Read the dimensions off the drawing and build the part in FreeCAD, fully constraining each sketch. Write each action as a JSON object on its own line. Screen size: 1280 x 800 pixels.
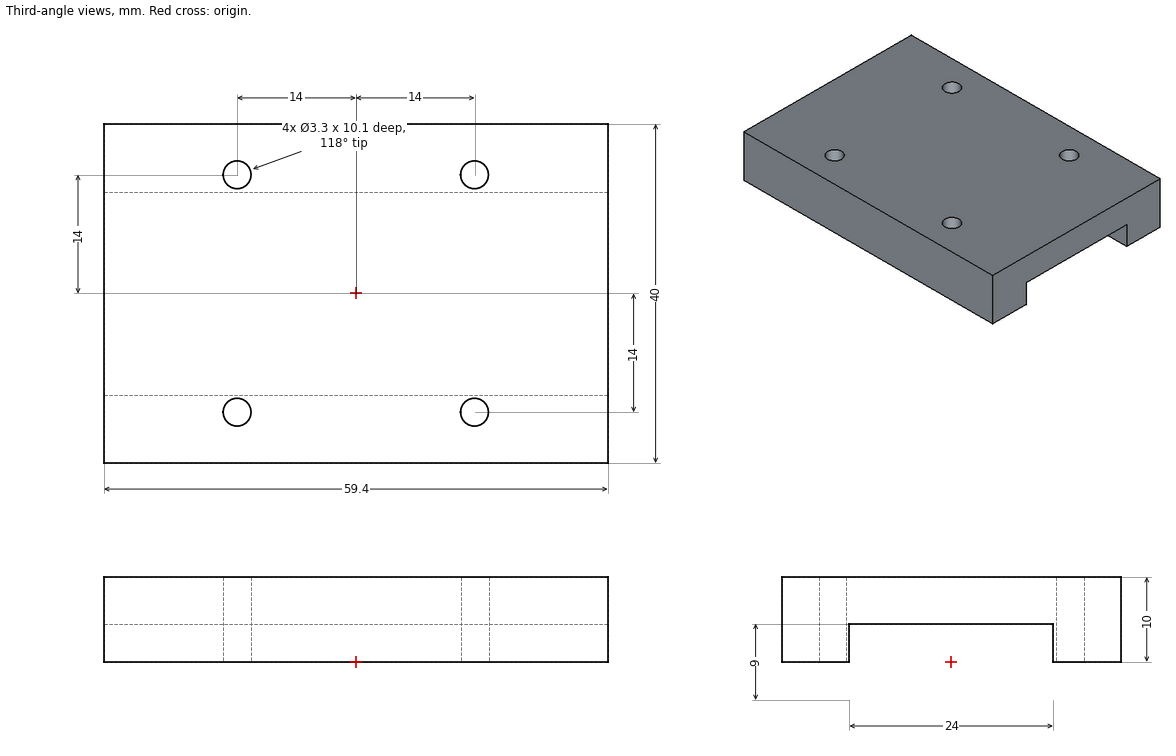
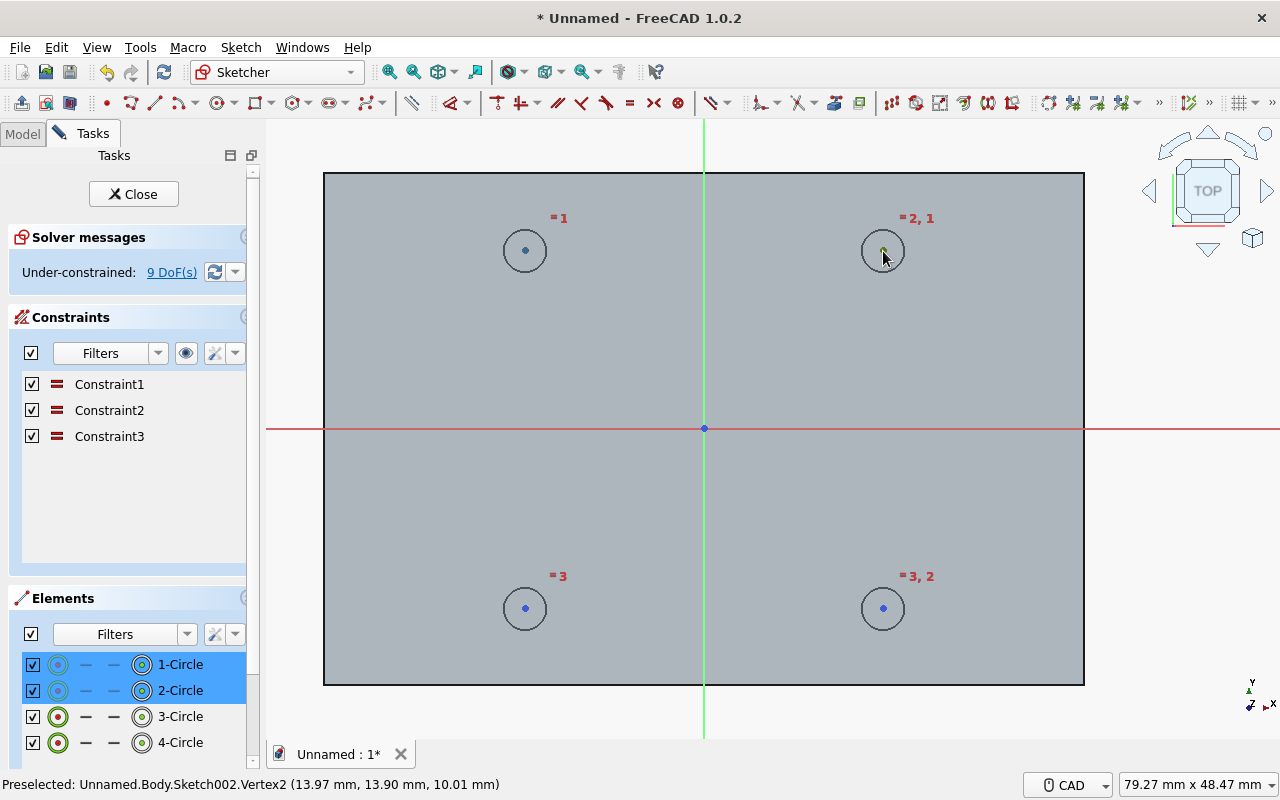
{"action": "key", "text": "h"}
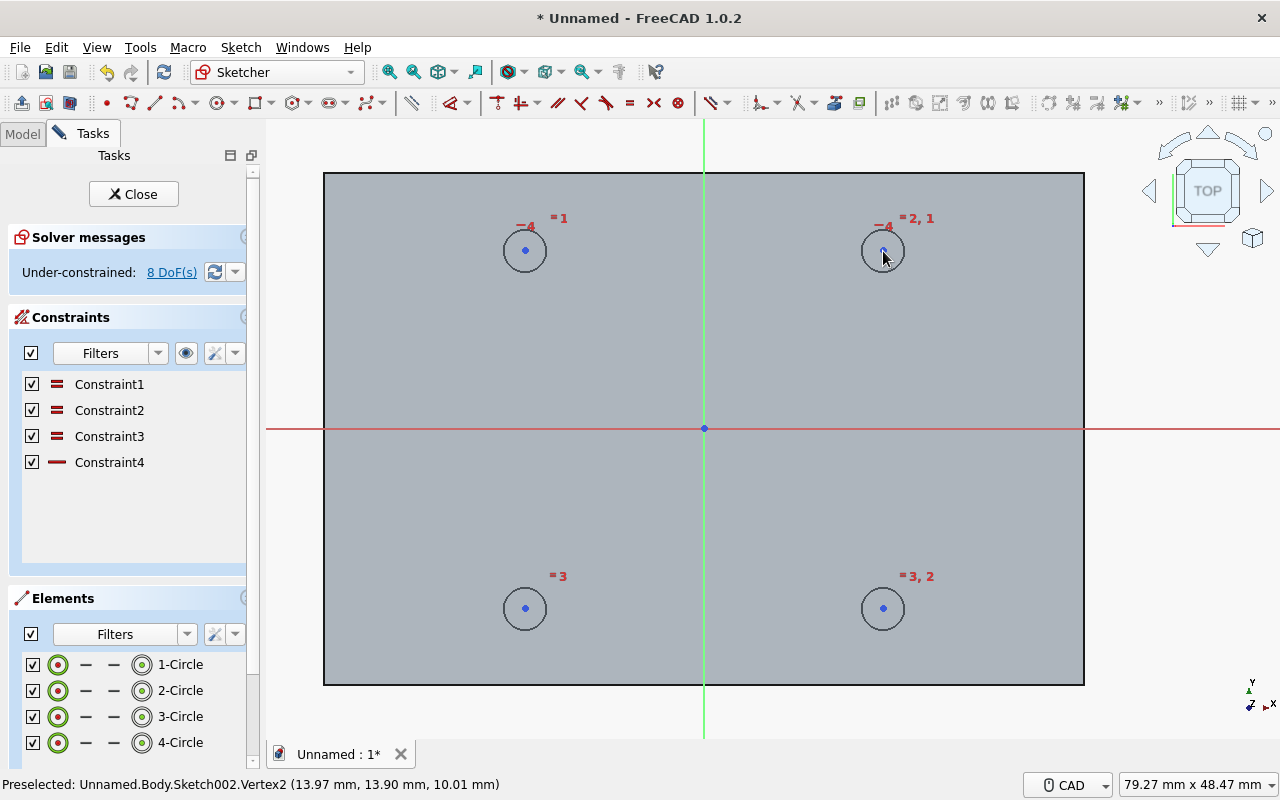
{"action": "left_click", "coordinate": [883, 251]}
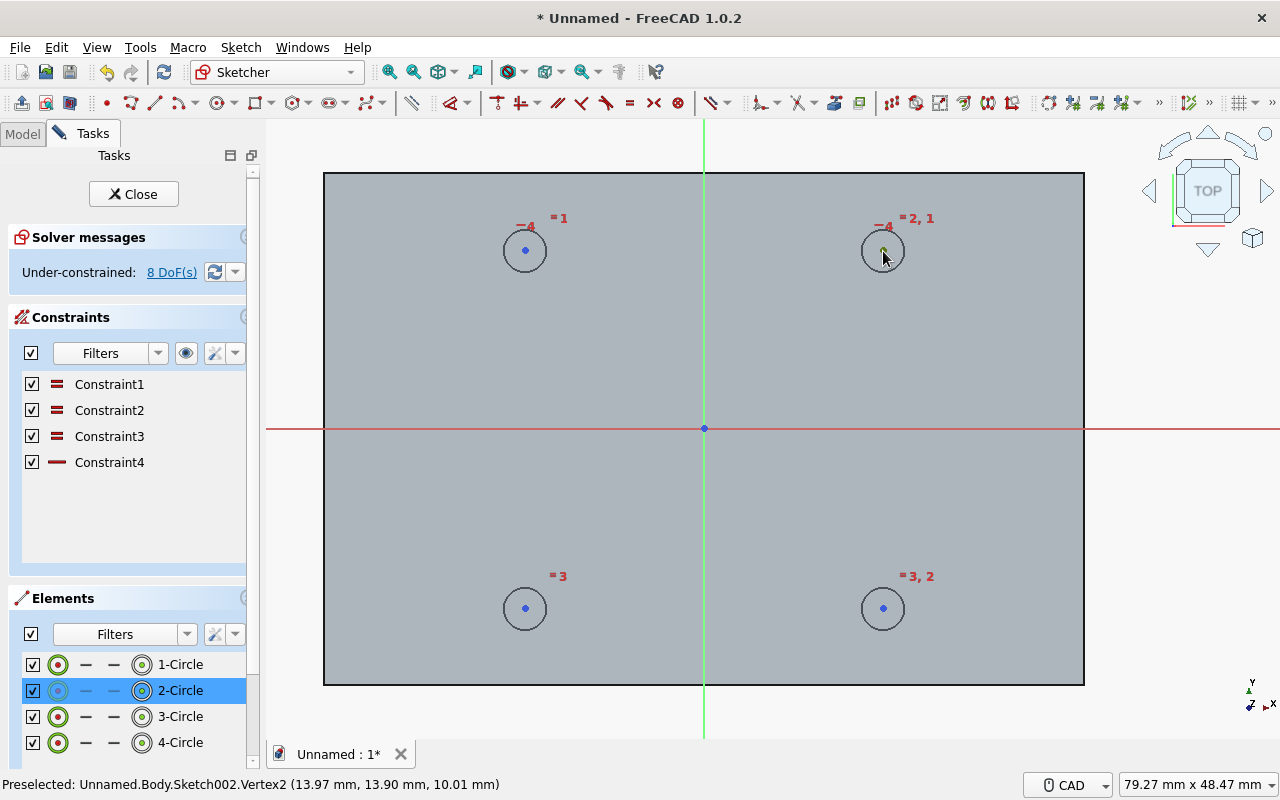
{"action": "left_click", "coordinate": [883, 609]}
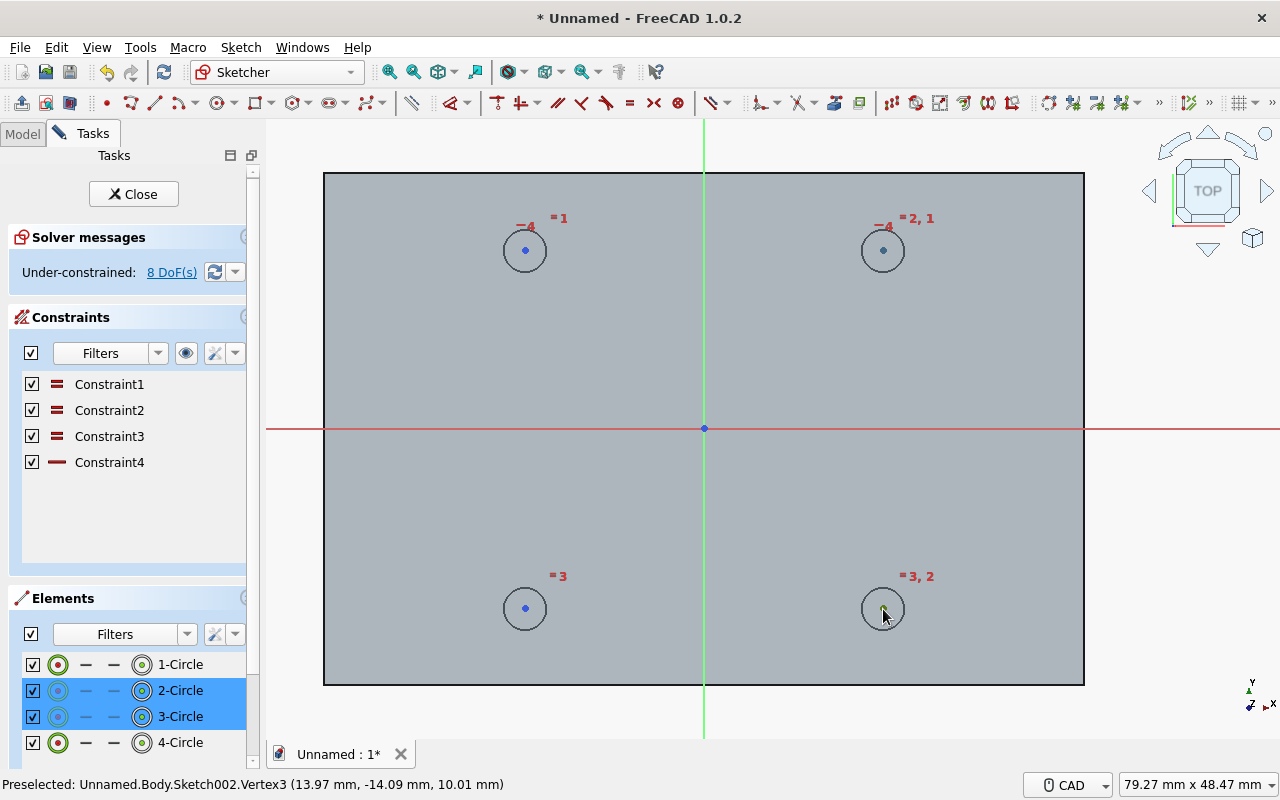
{"action": "key", "text": "v"}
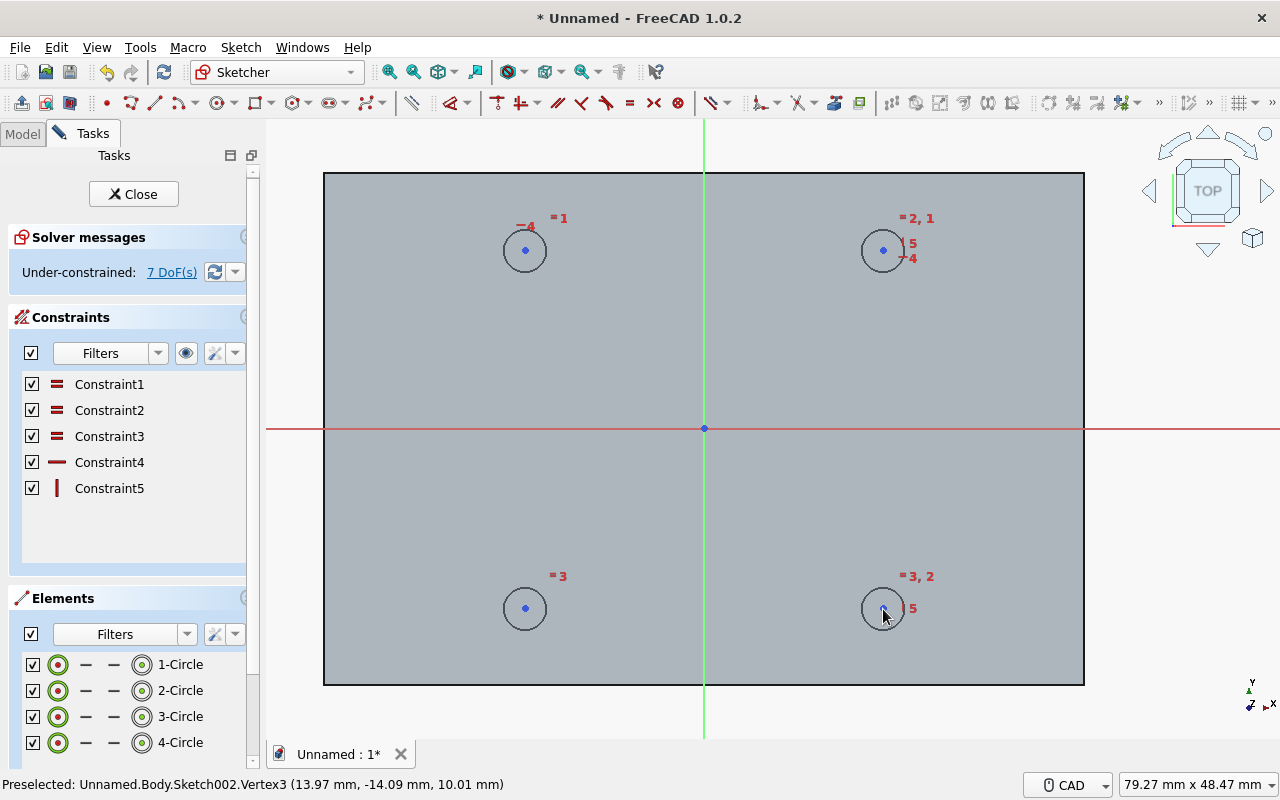
{"action": "left_click", "coordinate": [525, 251]}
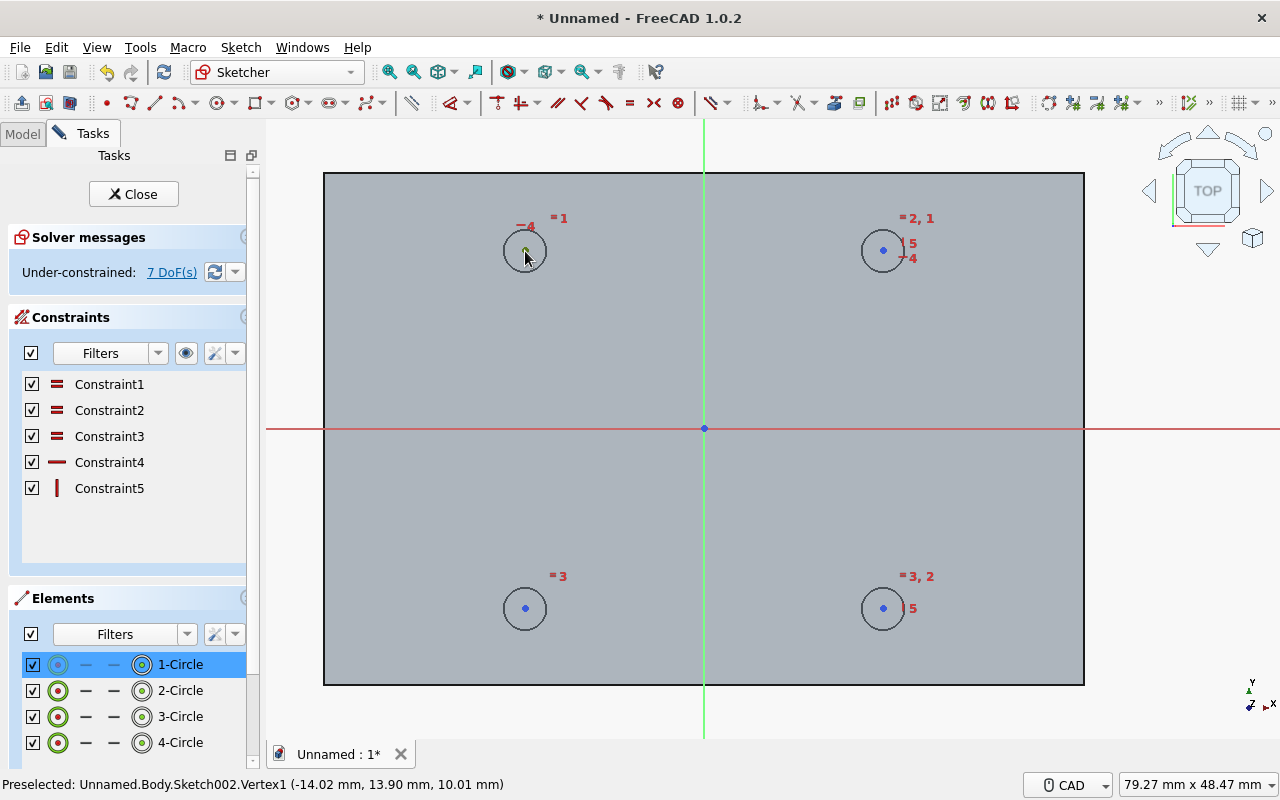
{"action": "left_click", "coordinate": [525, 609]}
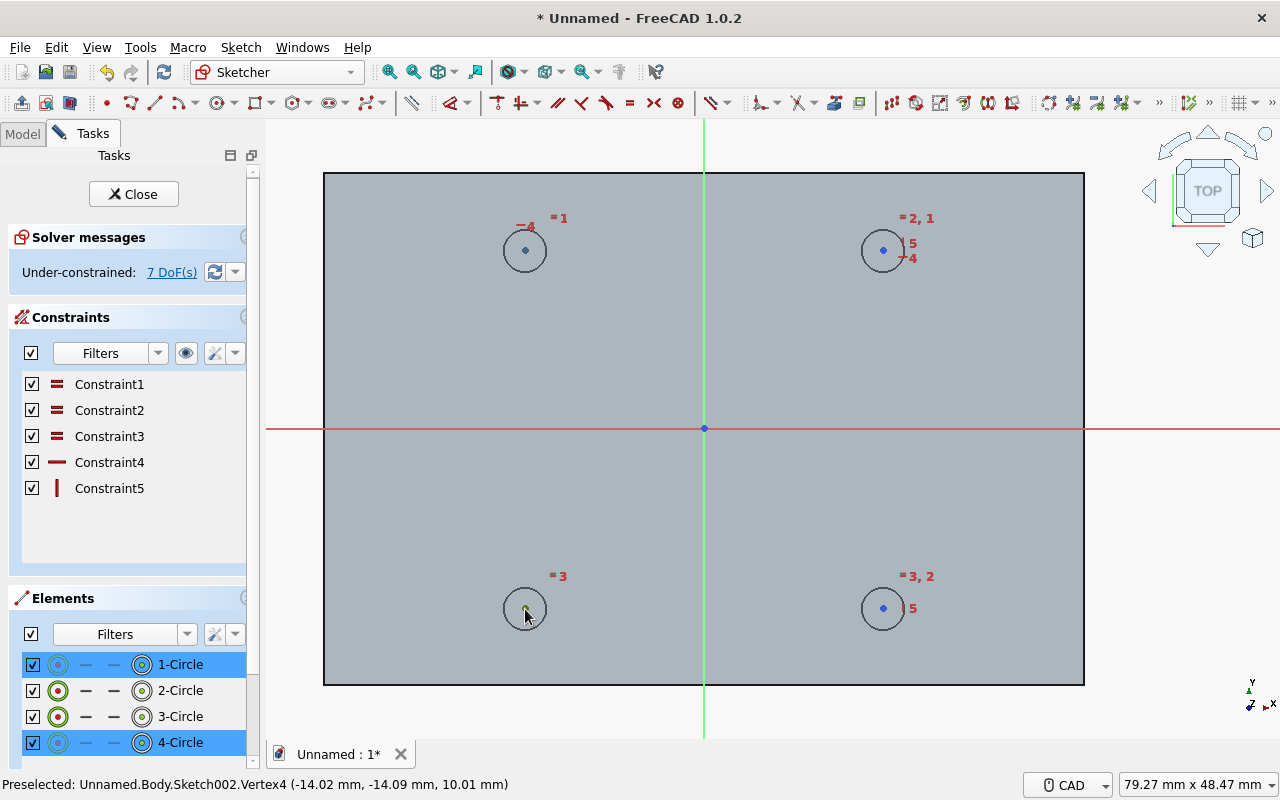
{"action": "key", "text": "v"}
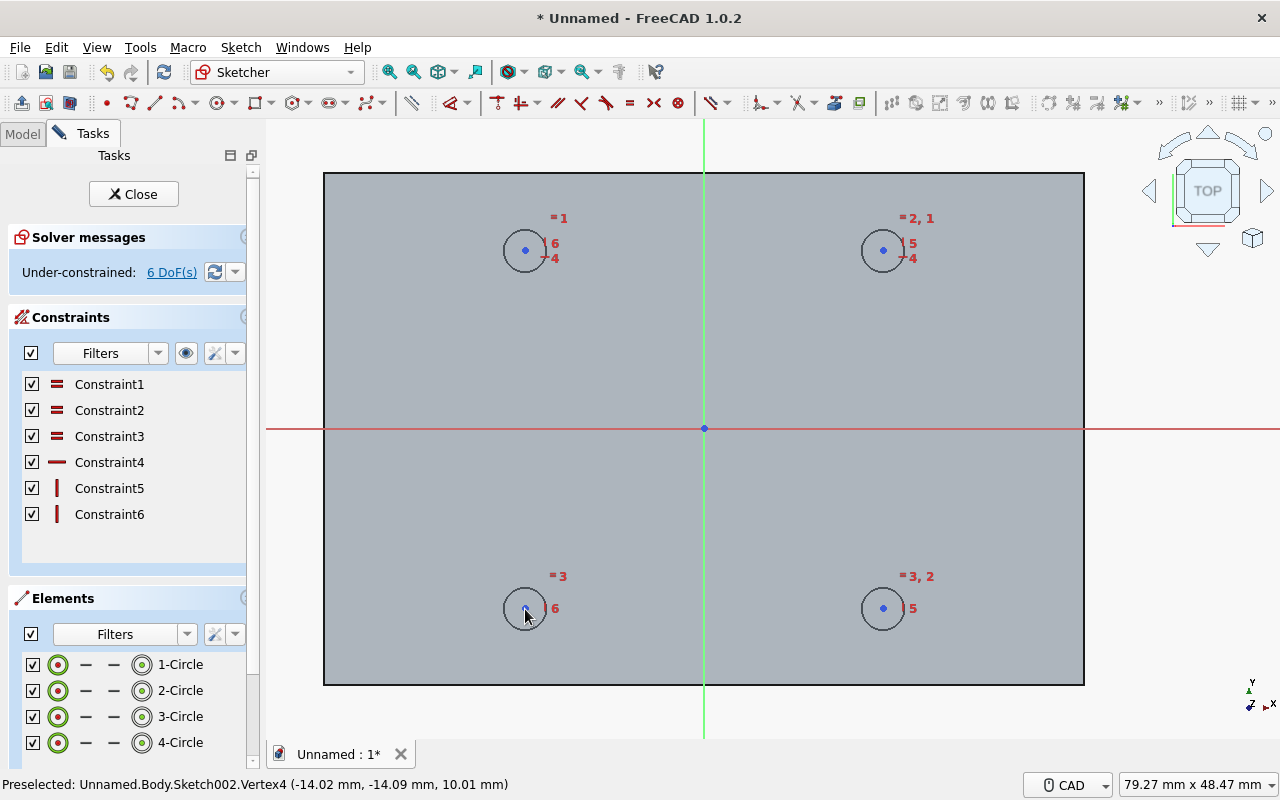
{"action": "left_click", "coordinate": [883, 609]}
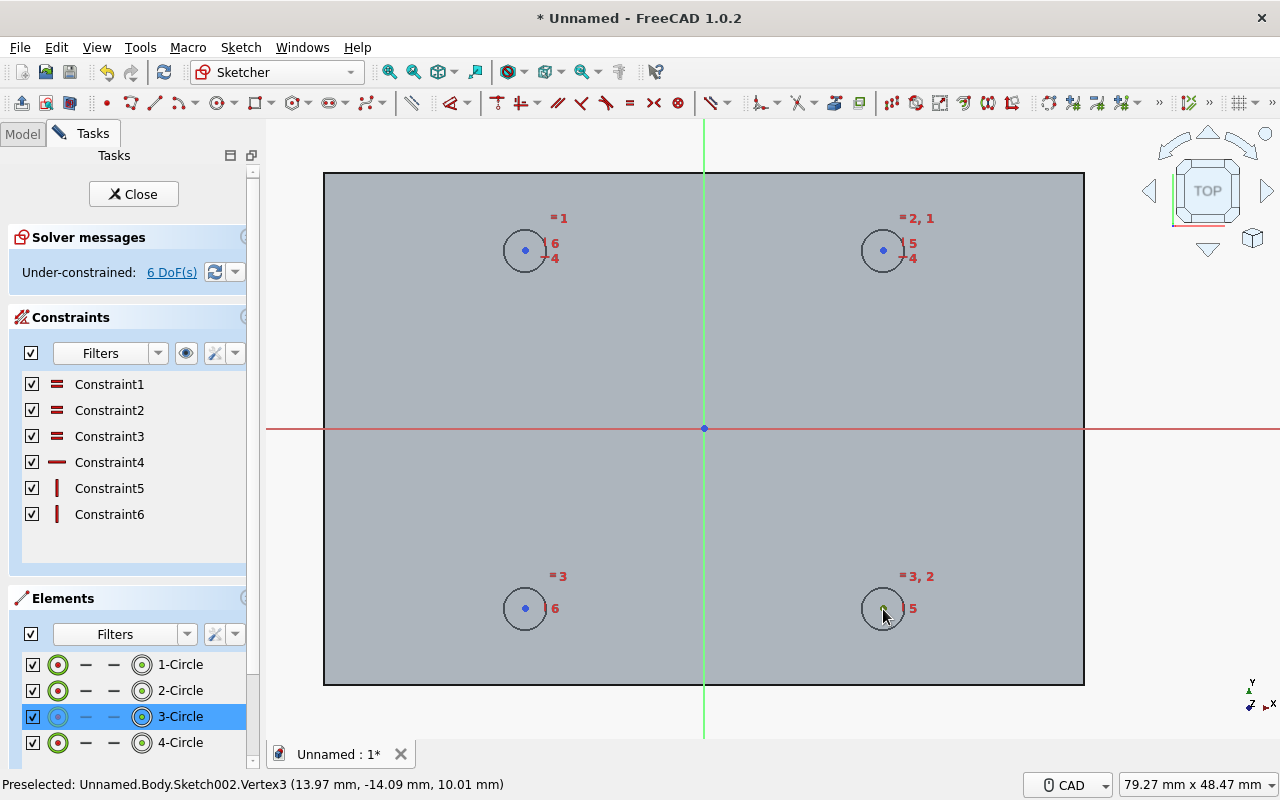
{"action": "left_click", "coordinate": [525, 609]}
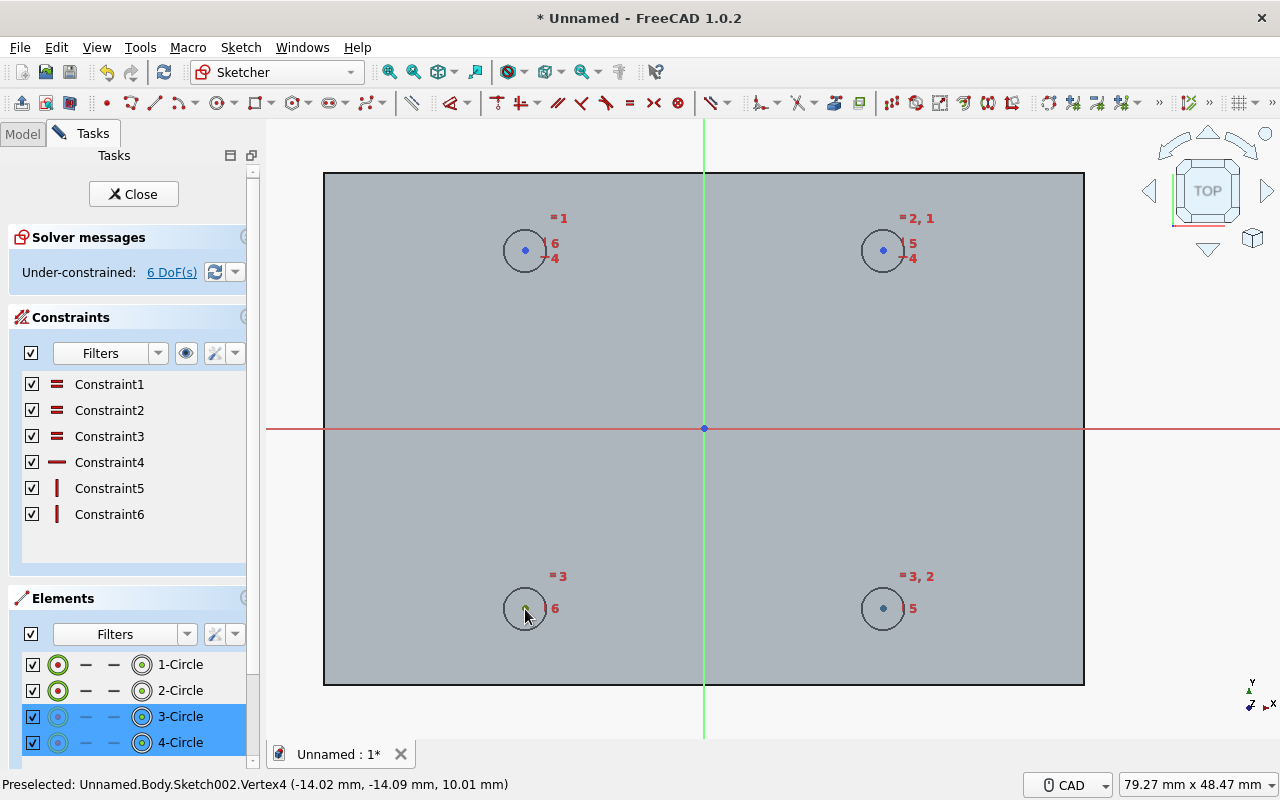
{"action": "key", "text": "h"}